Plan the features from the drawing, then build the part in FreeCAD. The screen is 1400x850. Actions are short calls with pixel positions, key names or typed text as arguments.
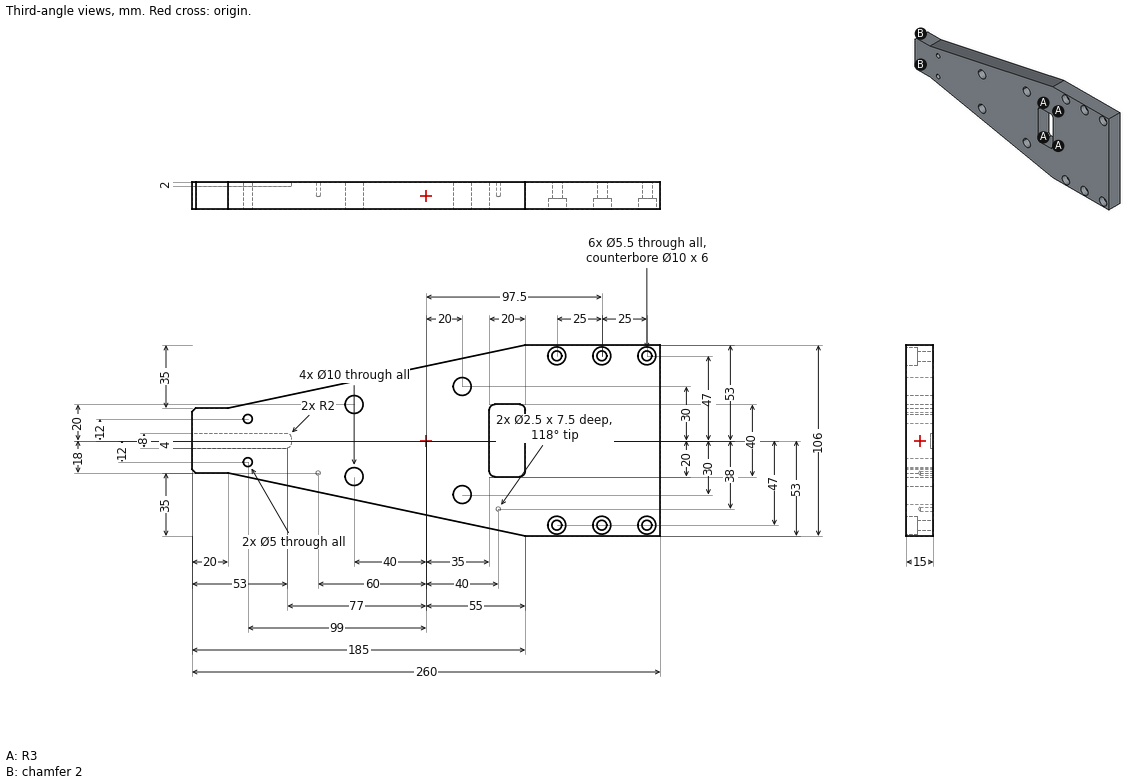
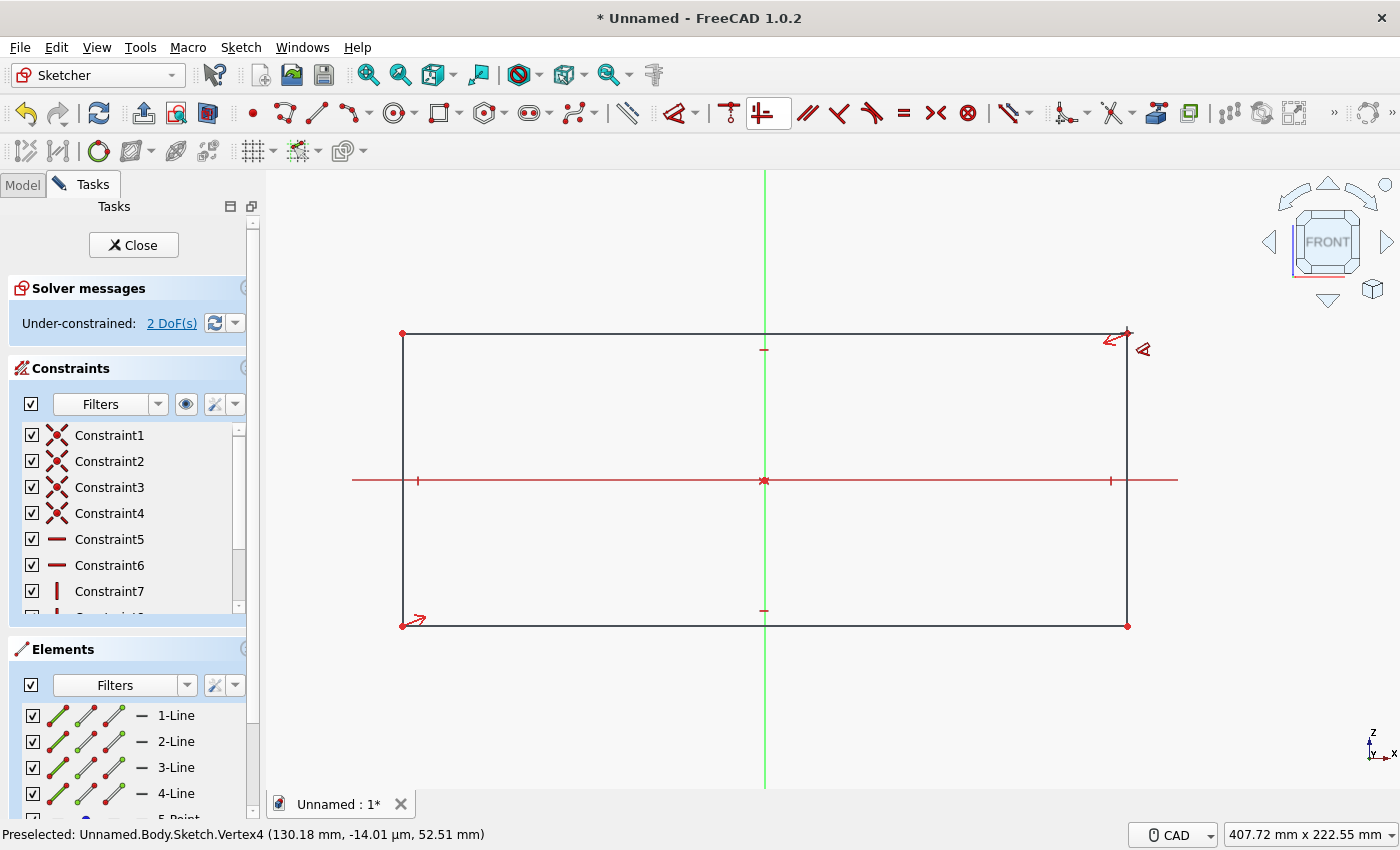
click(620, 626)
click(598, 660)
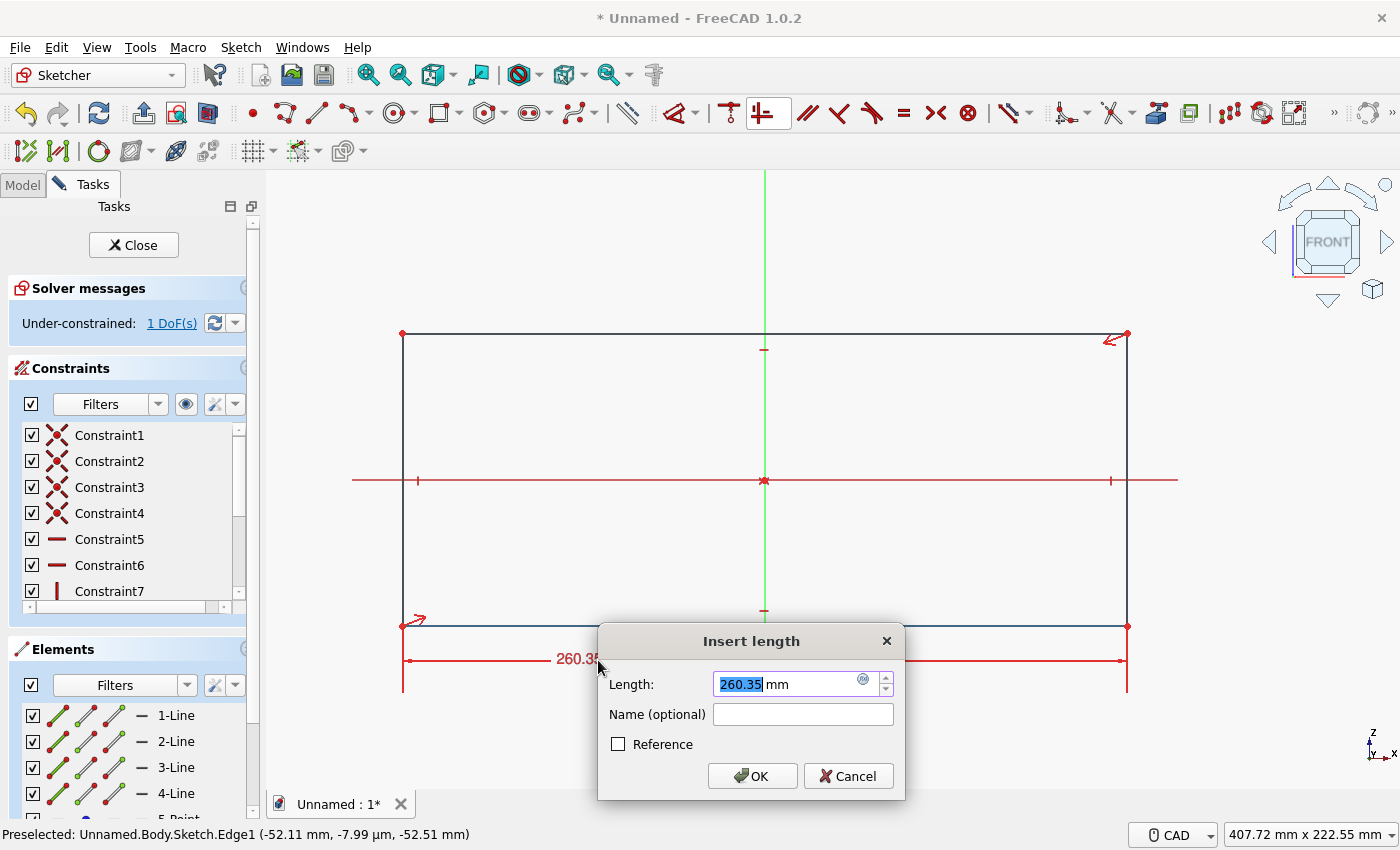
text(260)
key(Return)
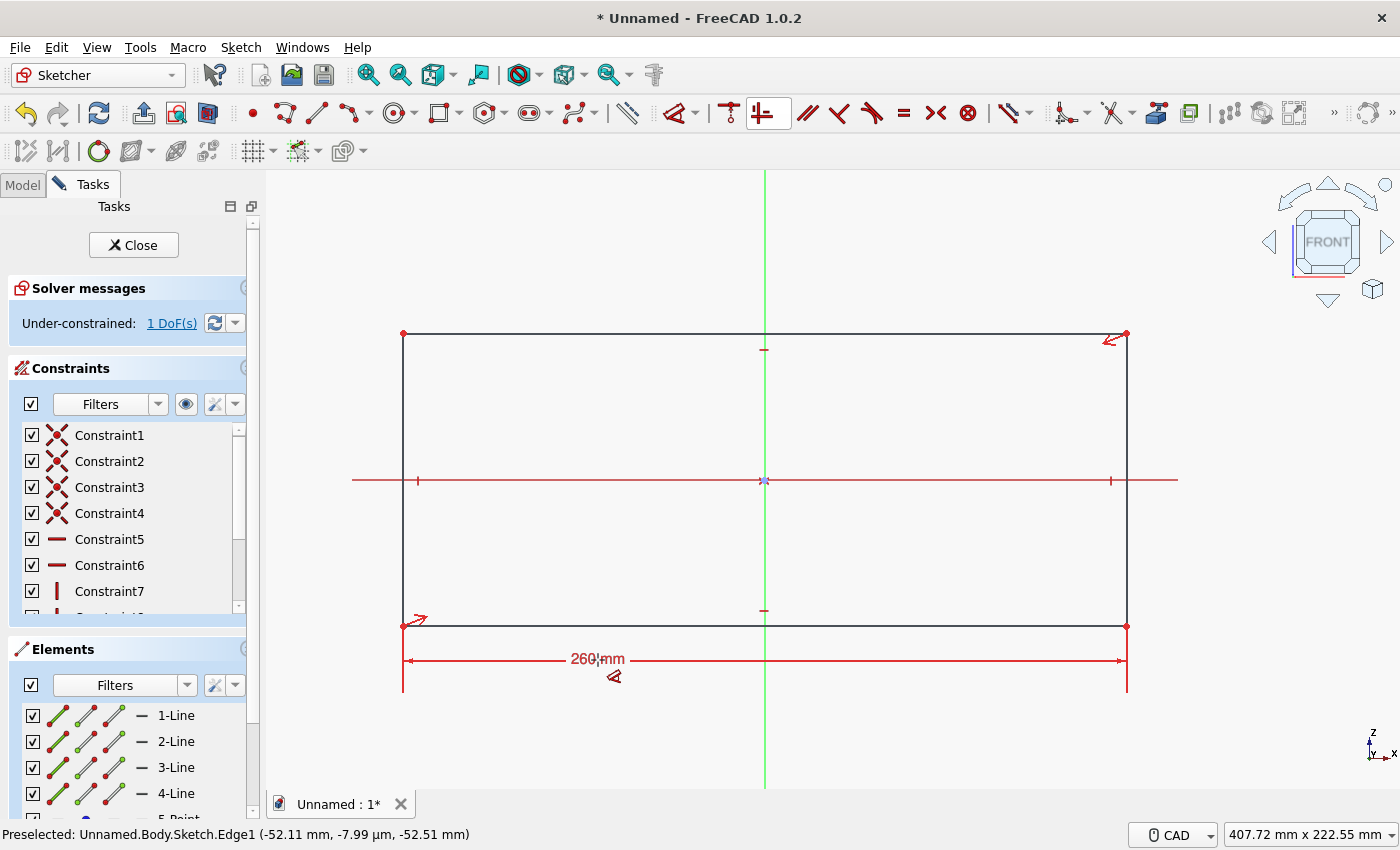
click(1127, 538)
click(1161, 413)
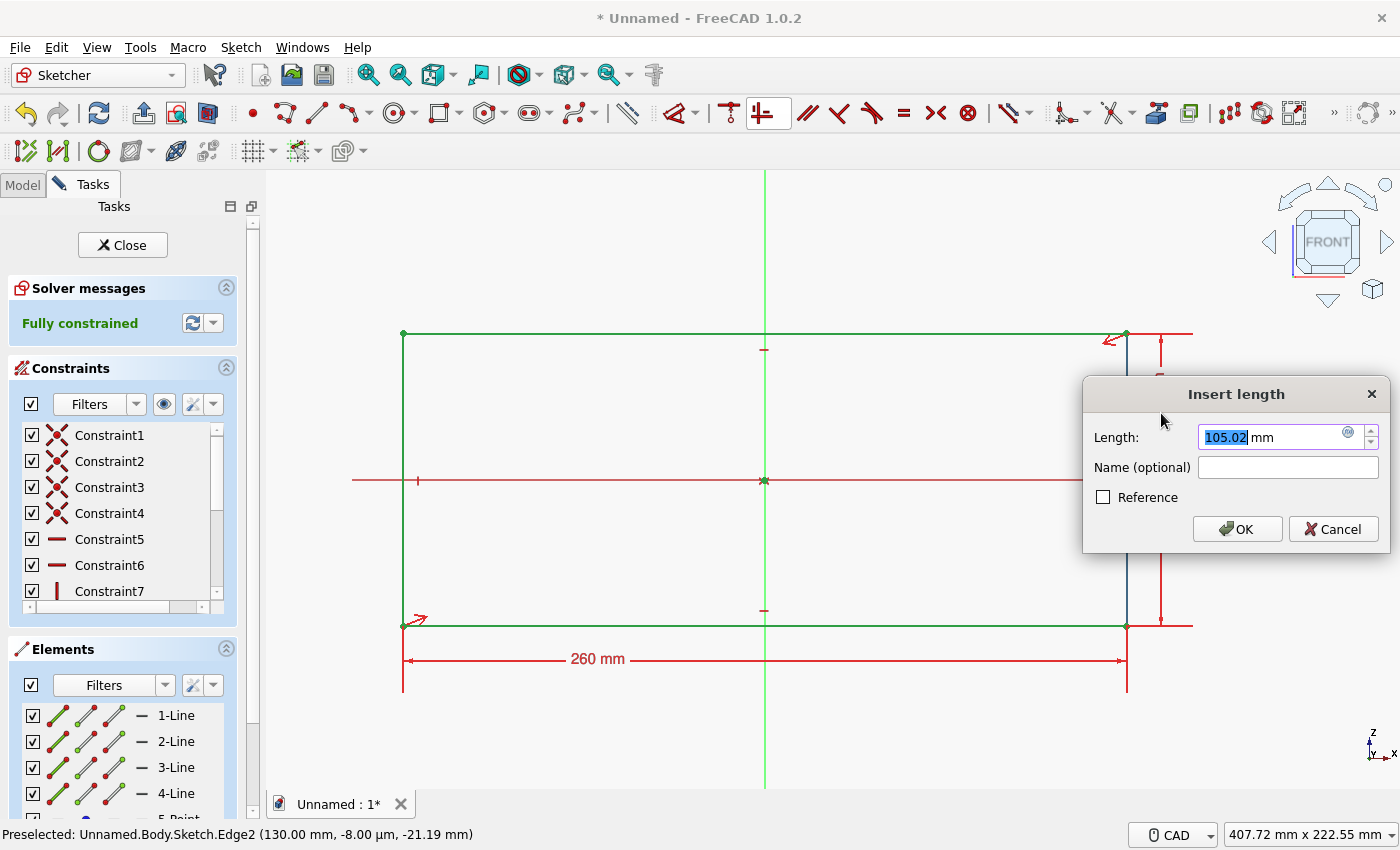
text(106)
key(Return)
key(Escape)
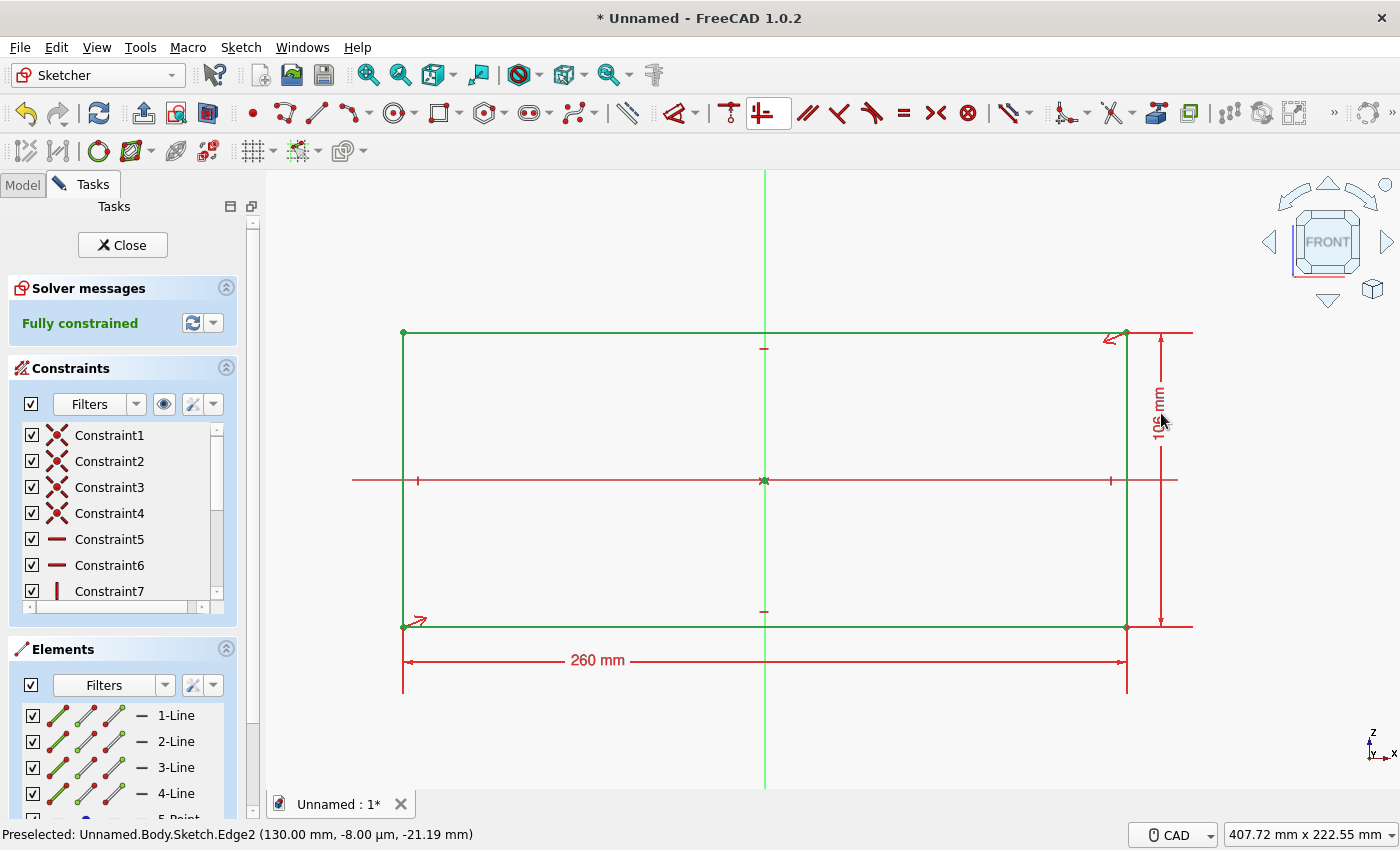
click(123, 245)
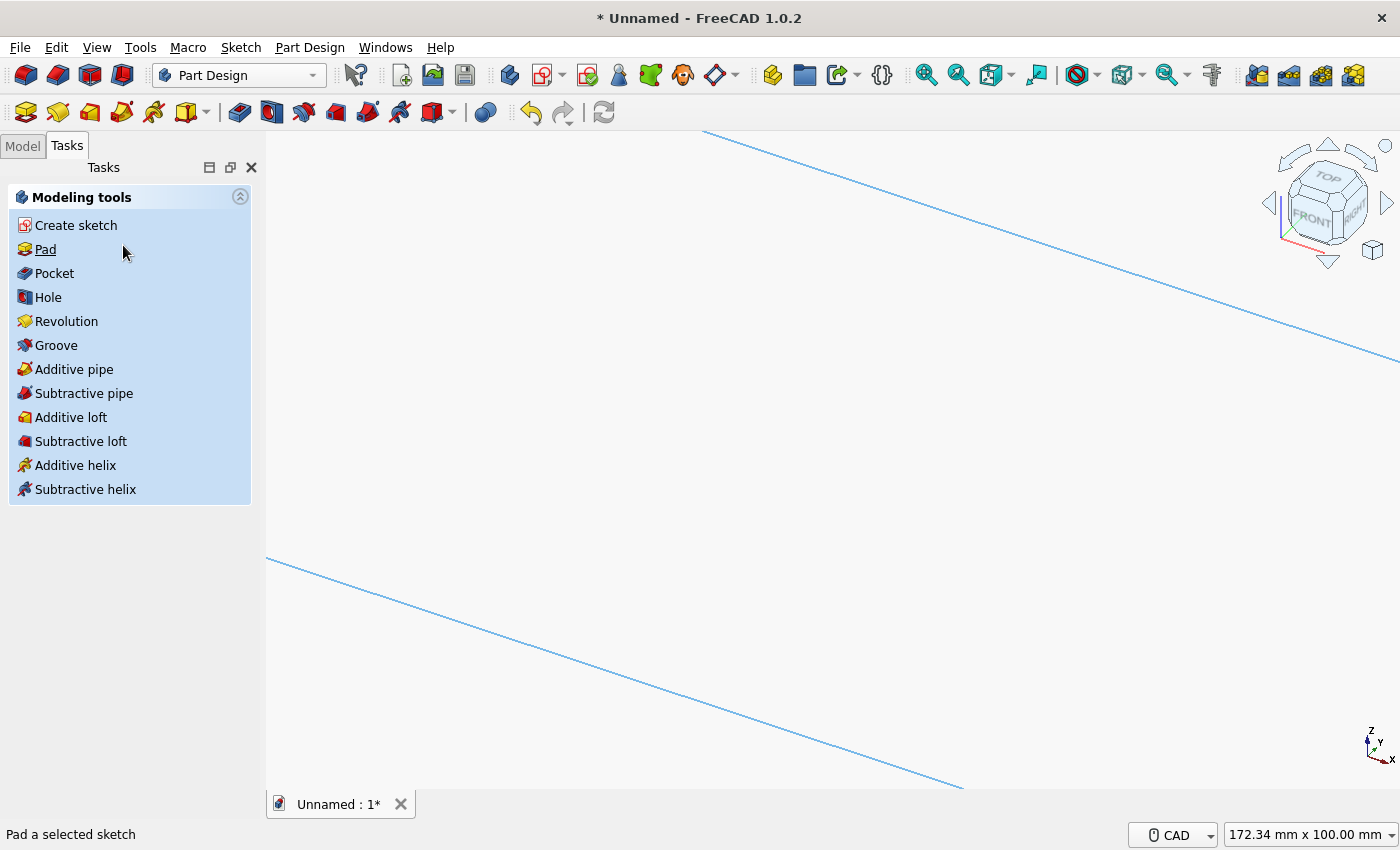
click(26, 112)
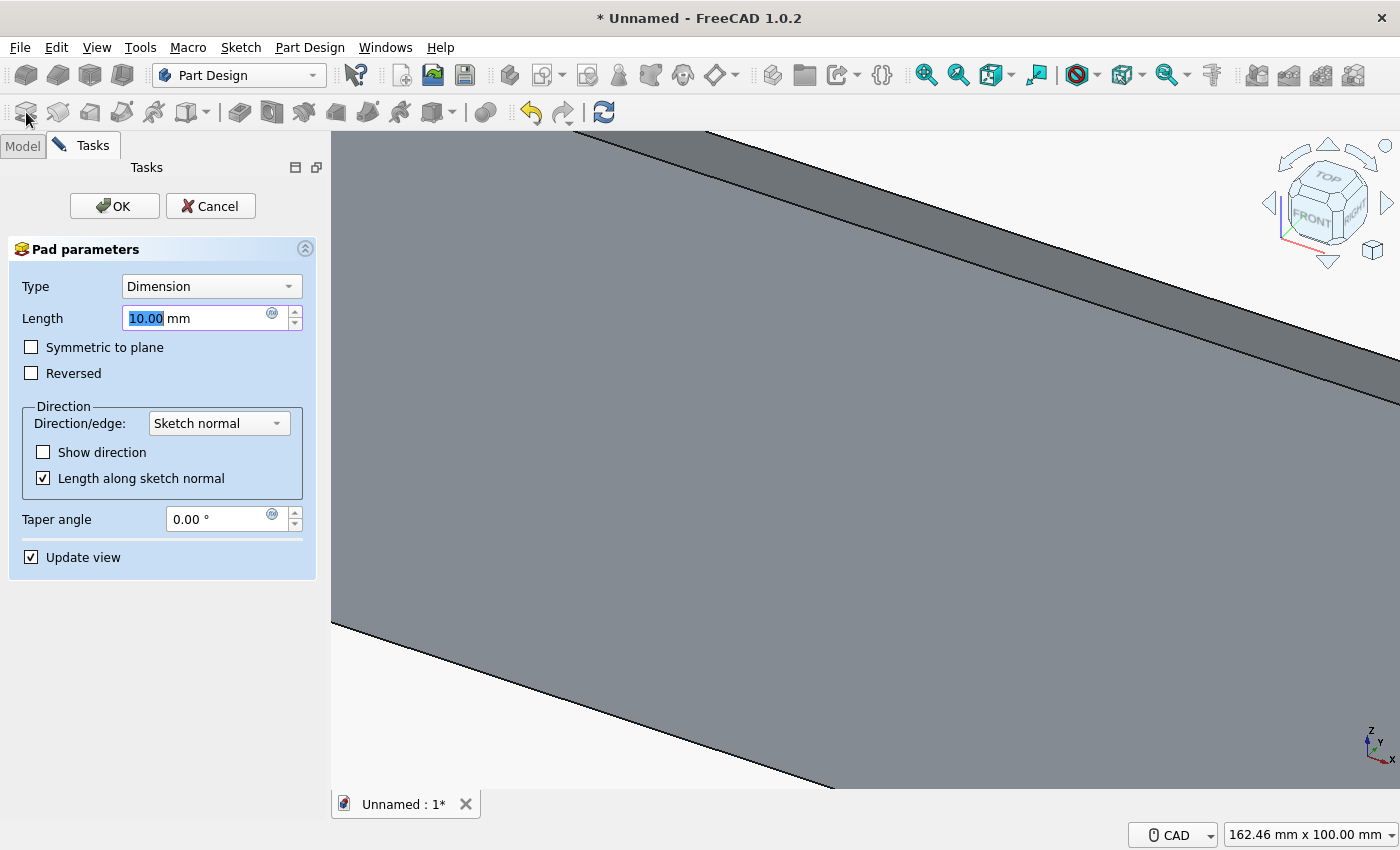
text(15)
key(Tab)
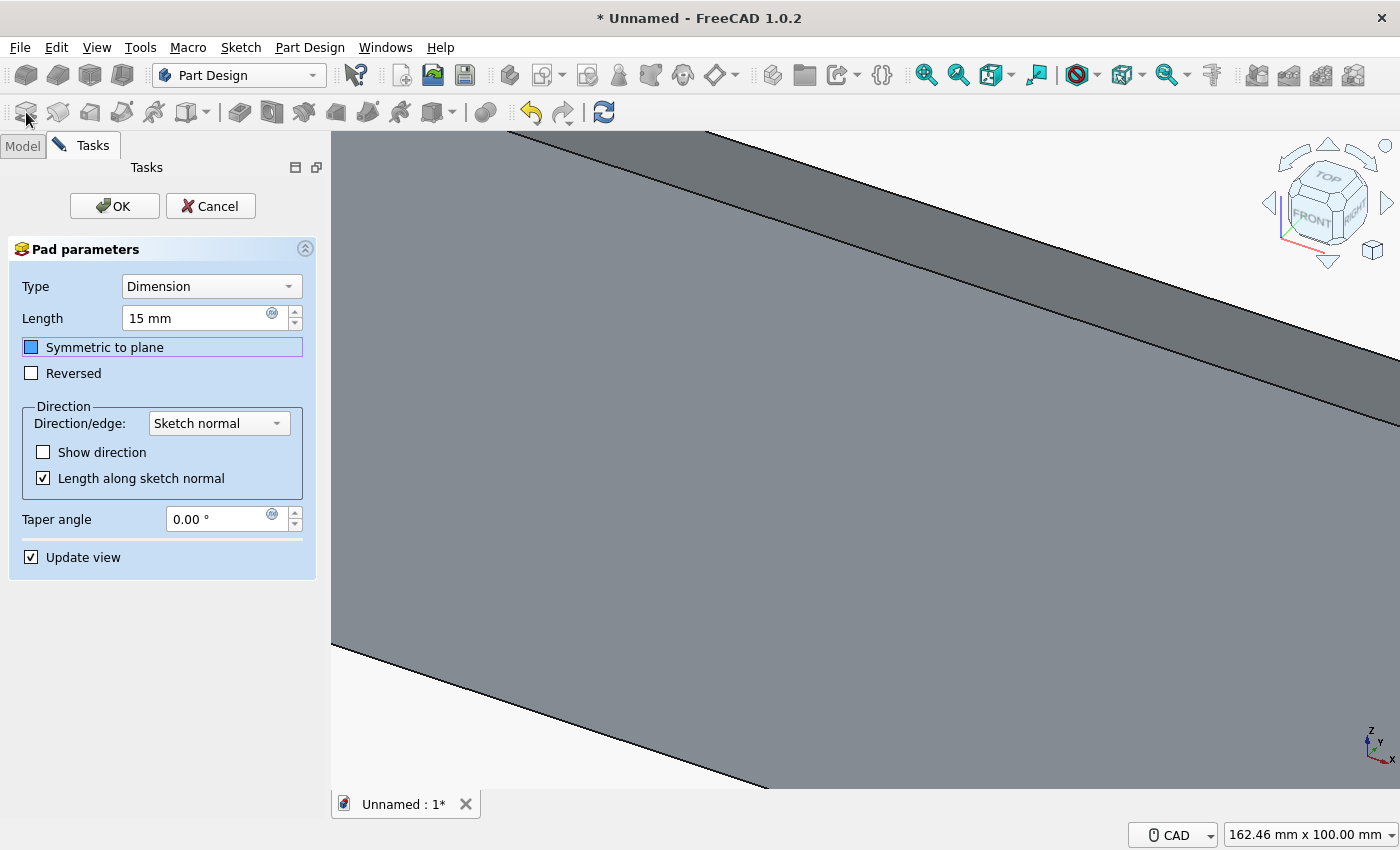
click(30, 347)